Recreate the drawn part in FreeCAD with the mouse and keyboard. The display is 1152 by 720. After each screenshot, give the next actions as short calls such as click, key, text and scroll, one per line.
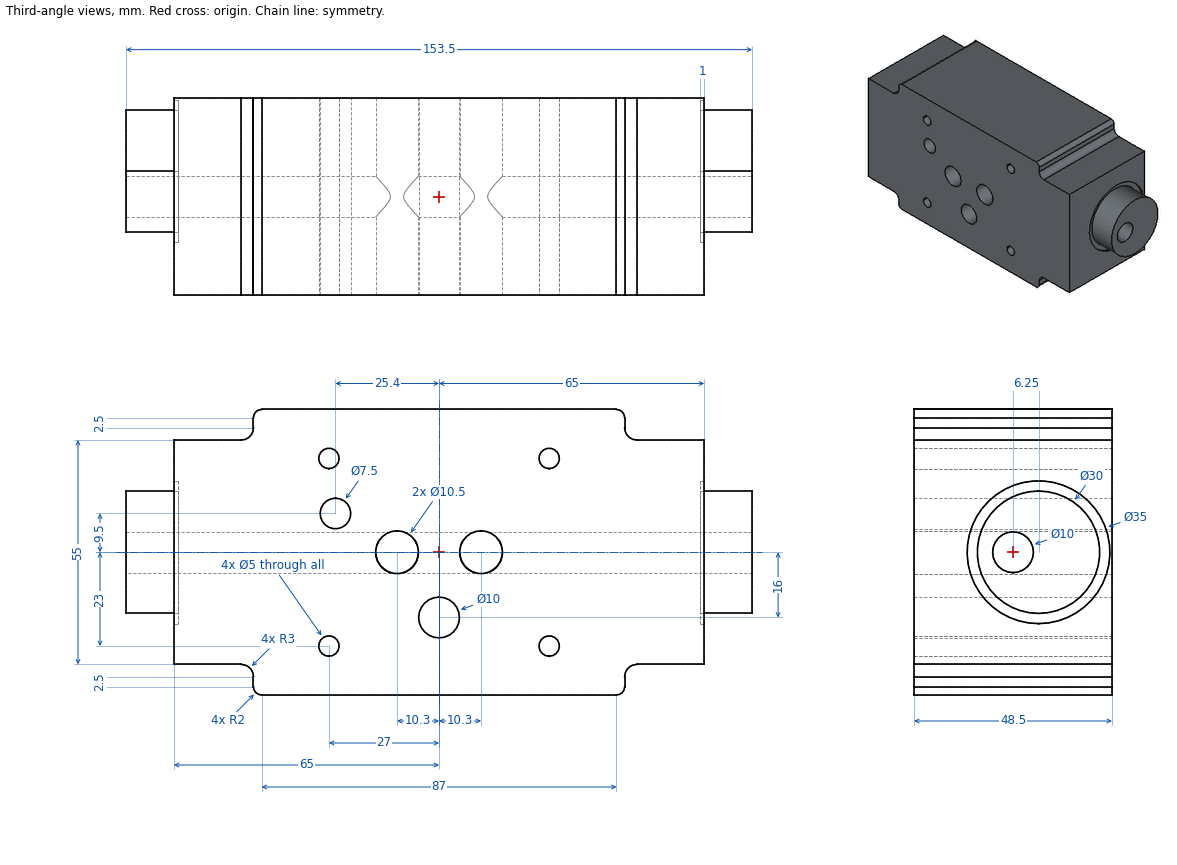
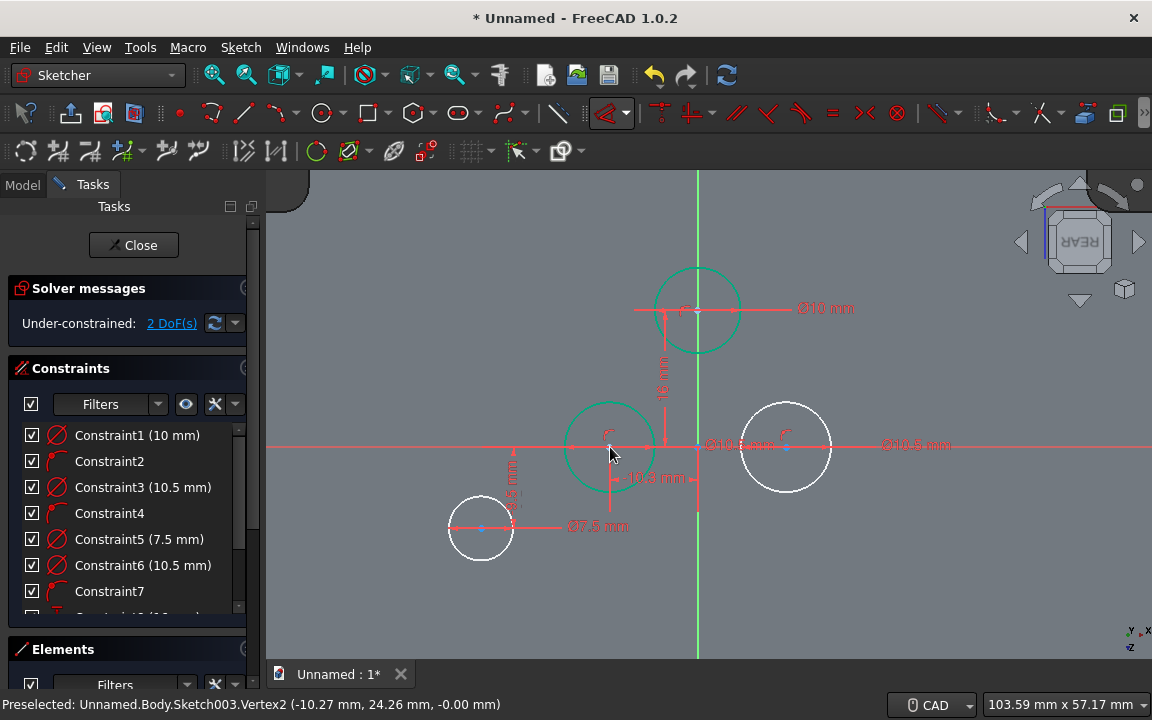
click(481, 528)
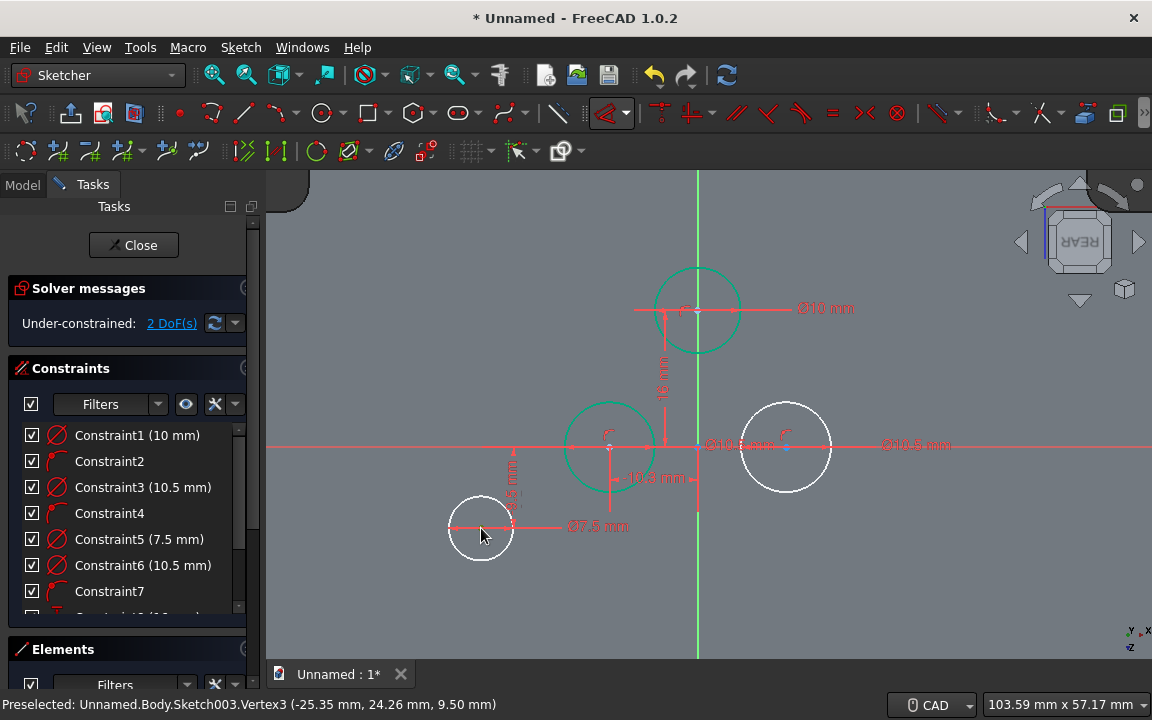
click(628, 114)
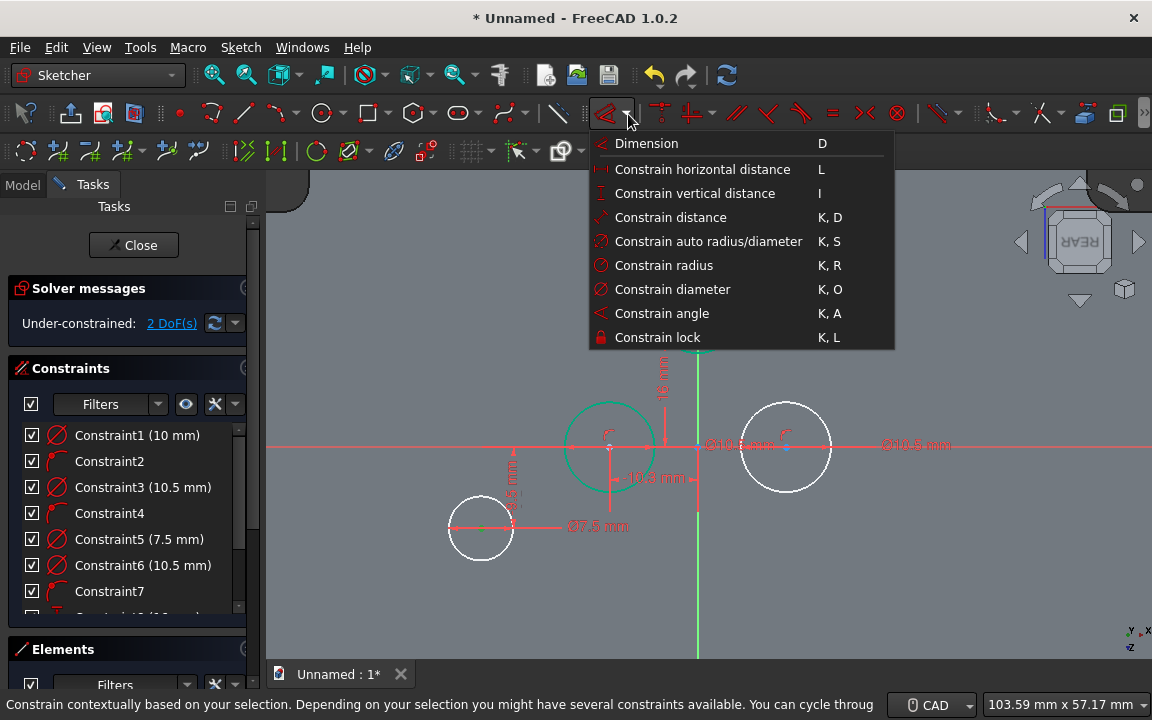
click(742, 169)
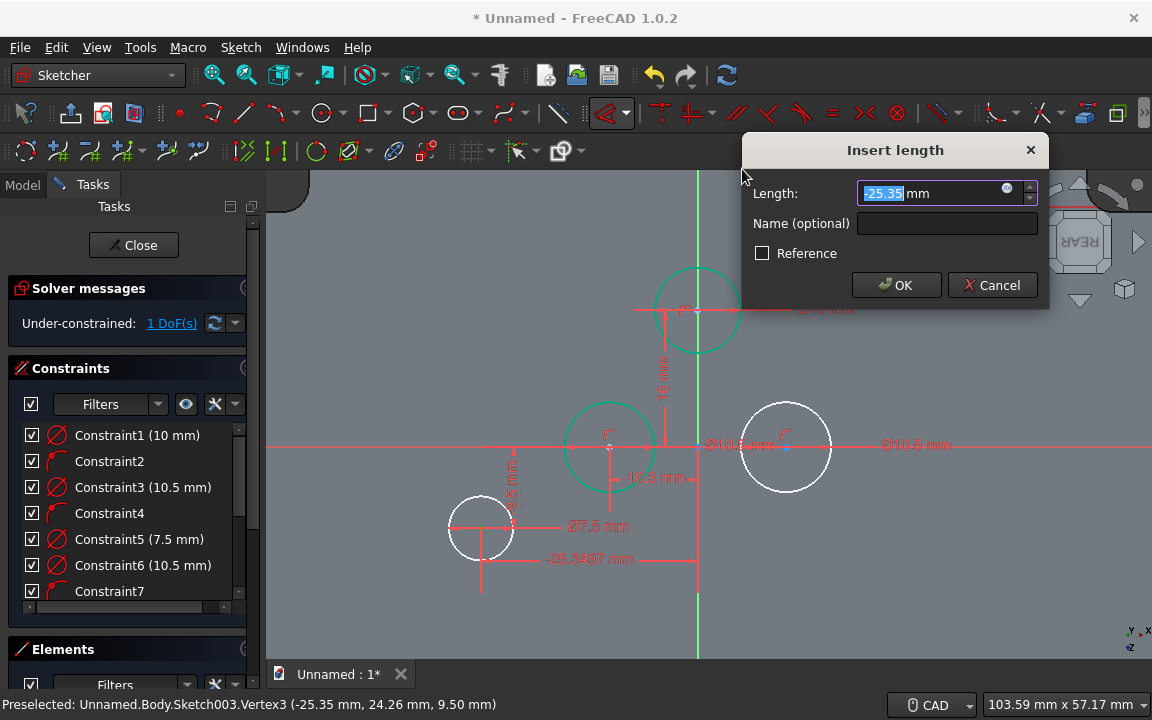
text(-25.4)
key(Return)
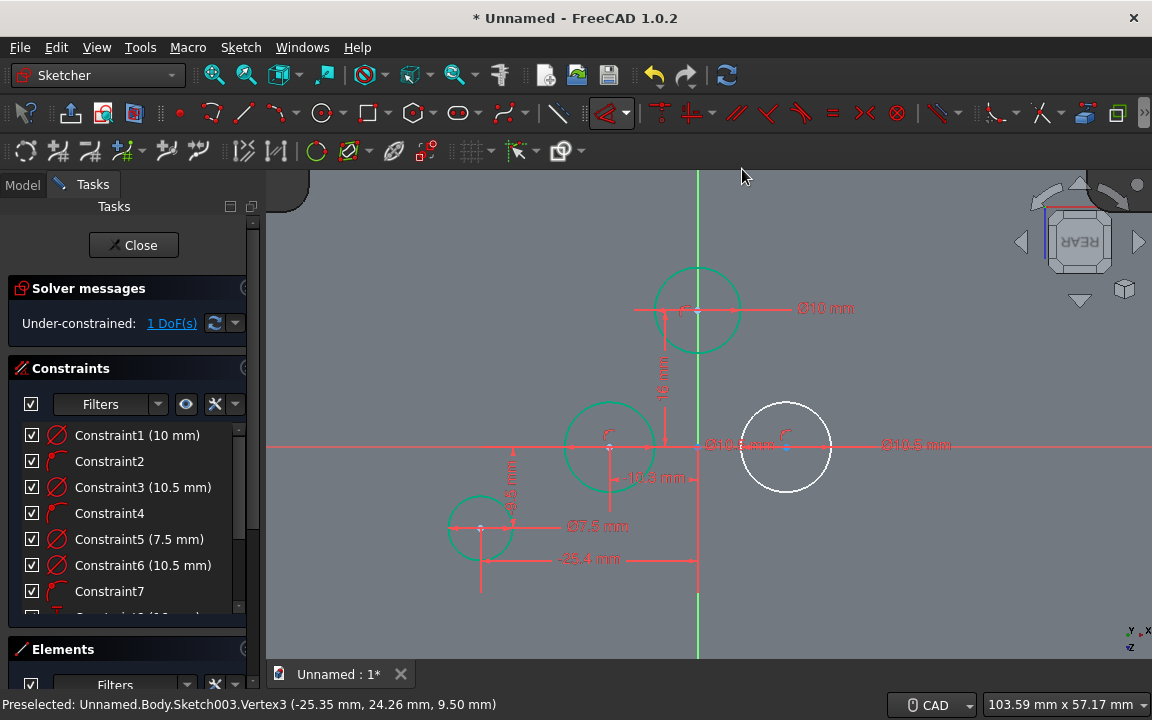
click(786, 447)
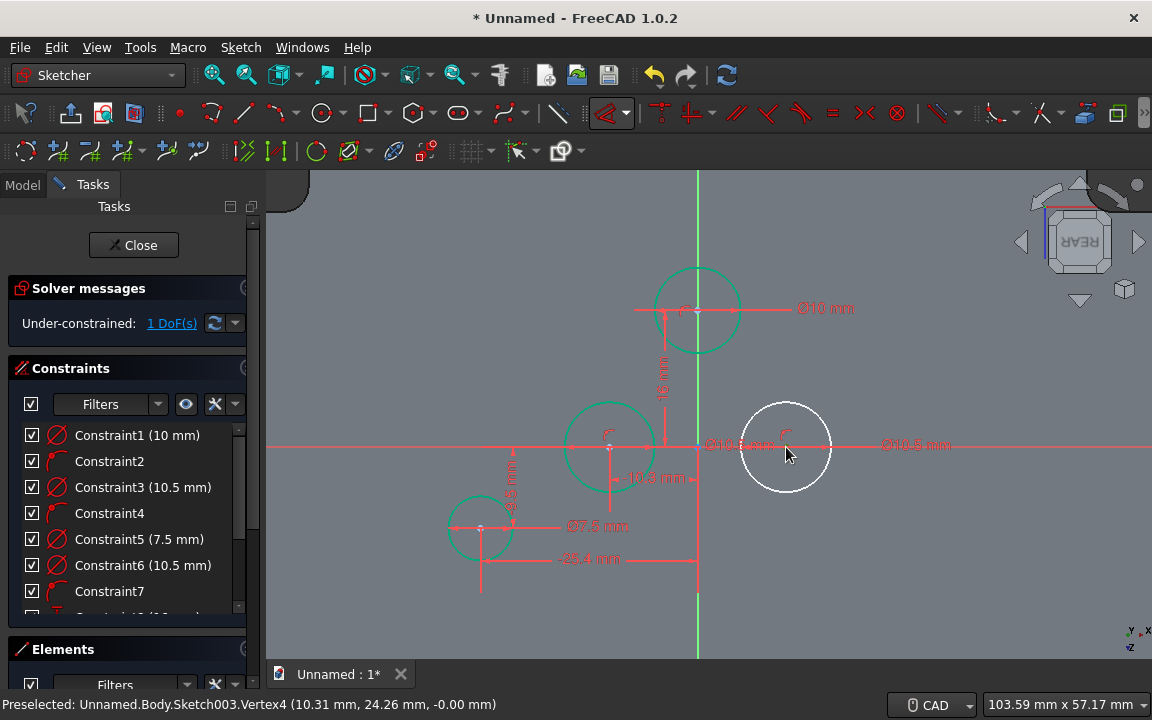
key(l)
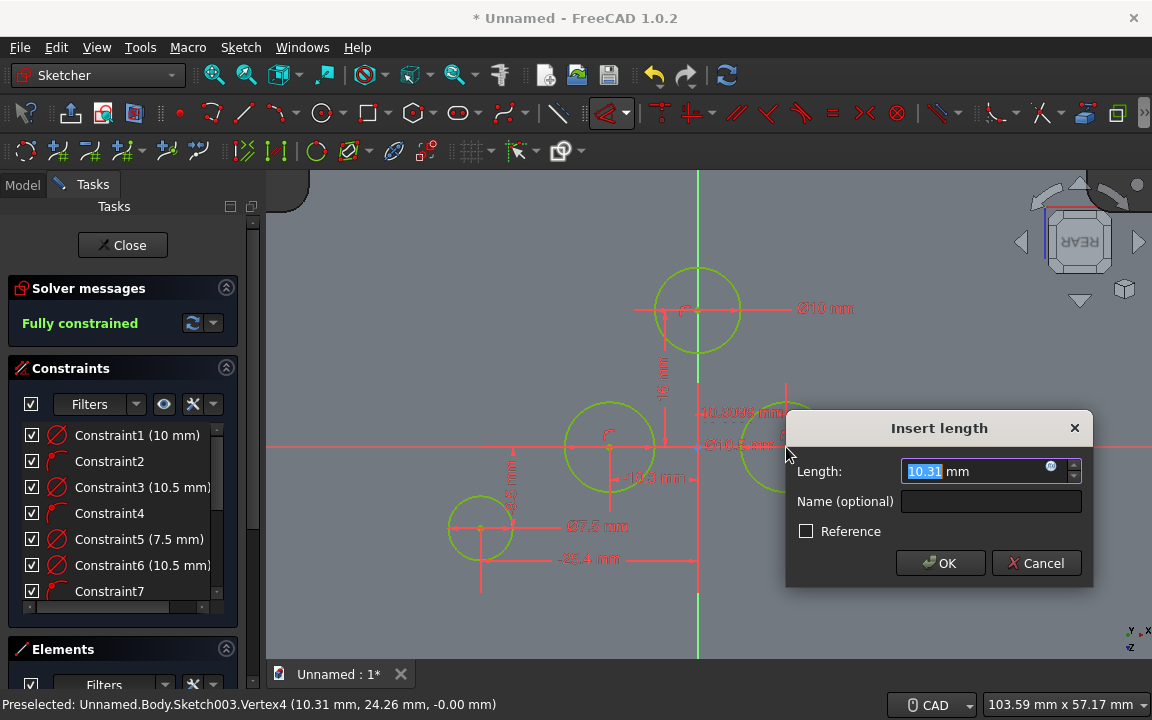
text(10.3)
key(Return)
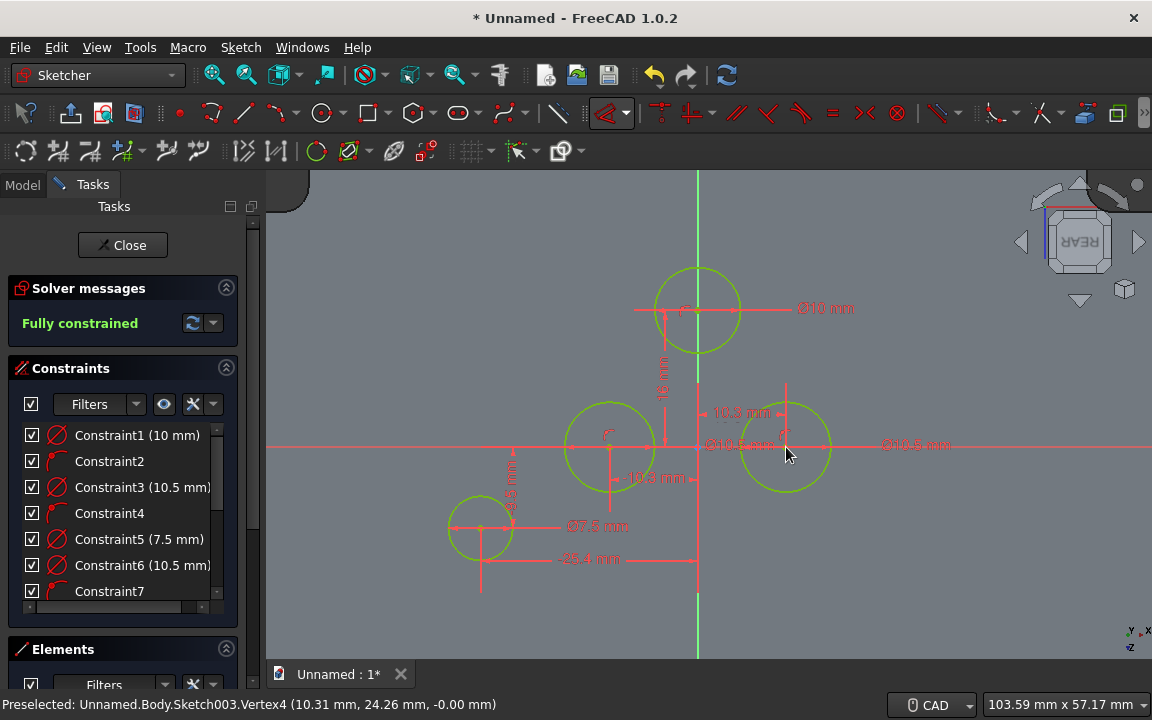
click(123, 245)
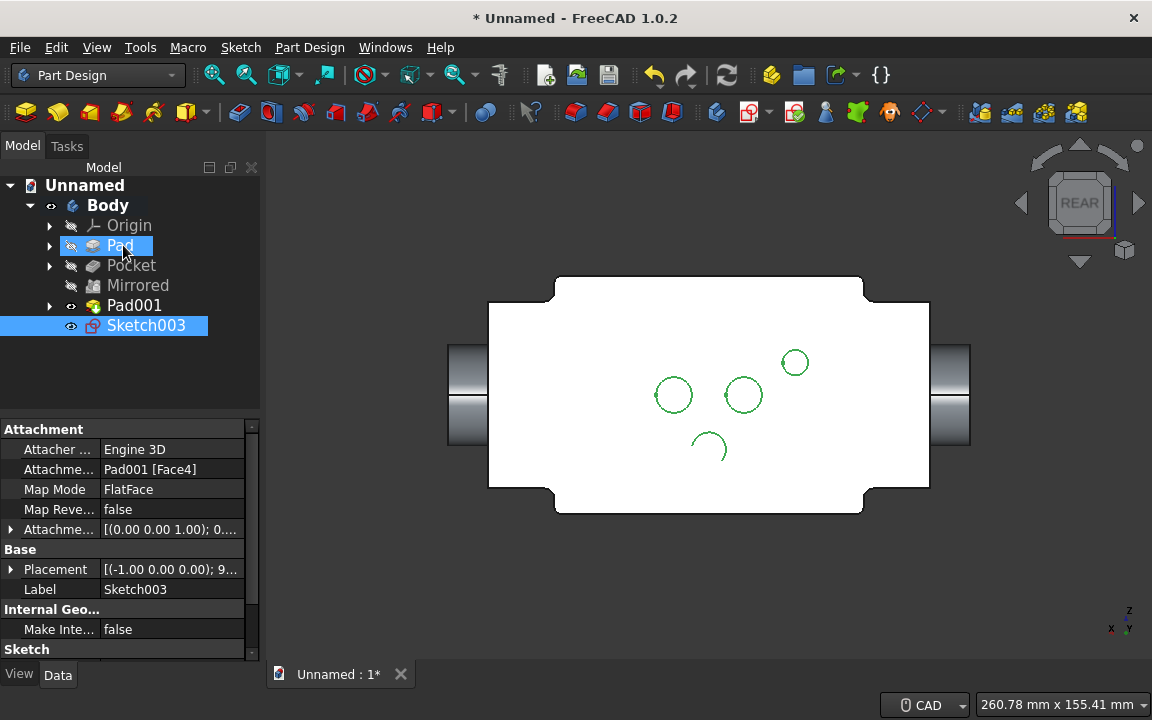
click(240, 112)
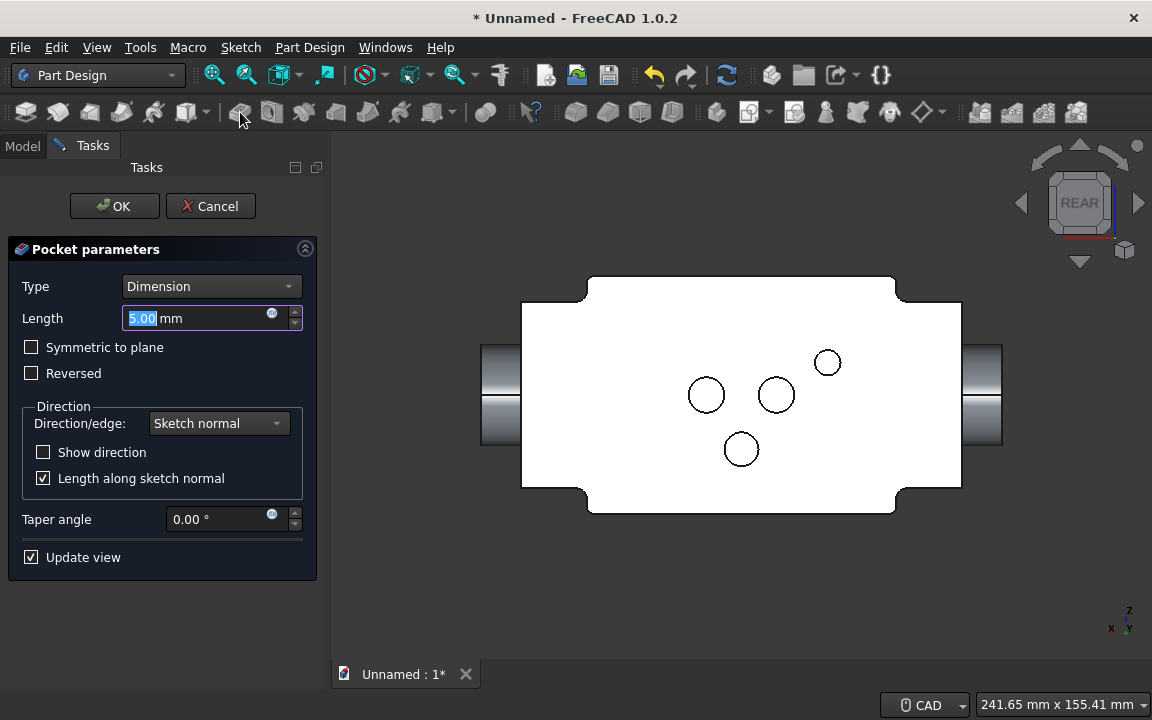
click(212, 286)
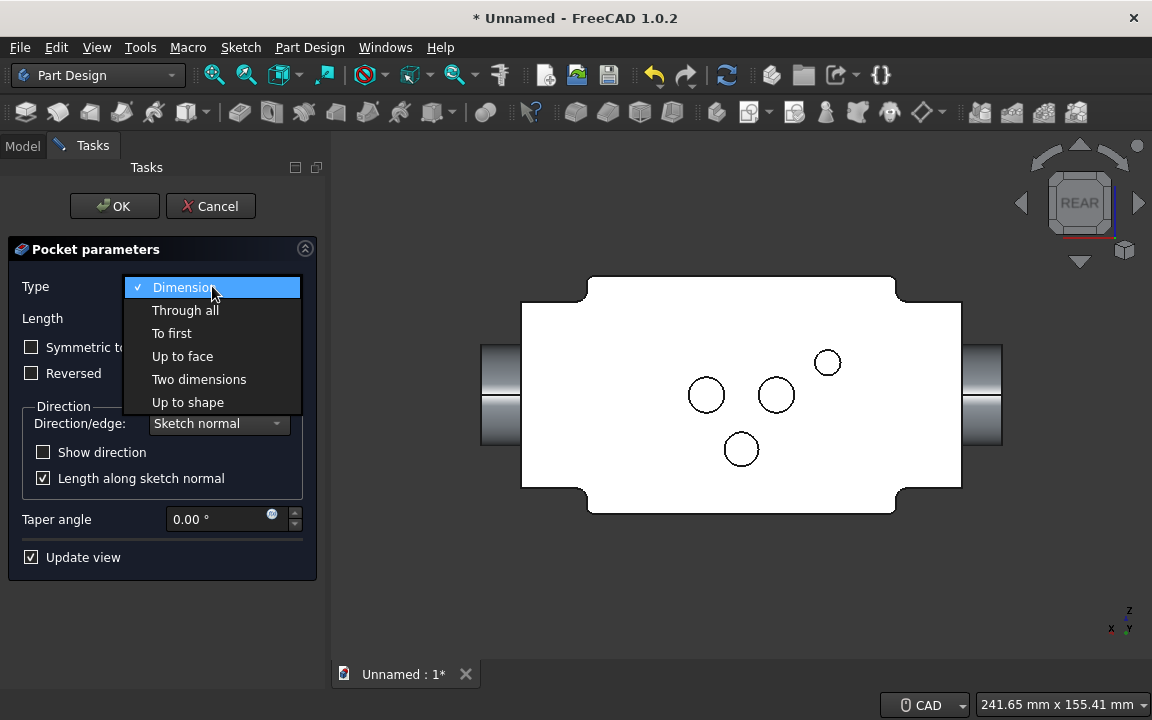
click(212, 310)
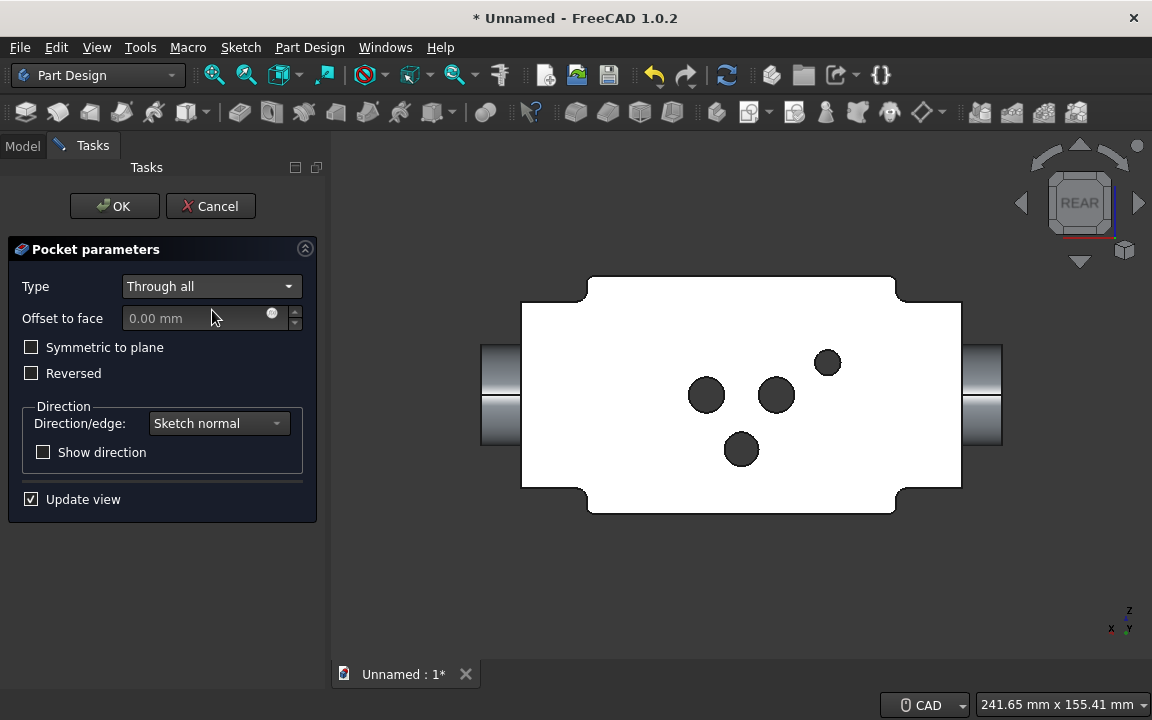
click(115, 206)